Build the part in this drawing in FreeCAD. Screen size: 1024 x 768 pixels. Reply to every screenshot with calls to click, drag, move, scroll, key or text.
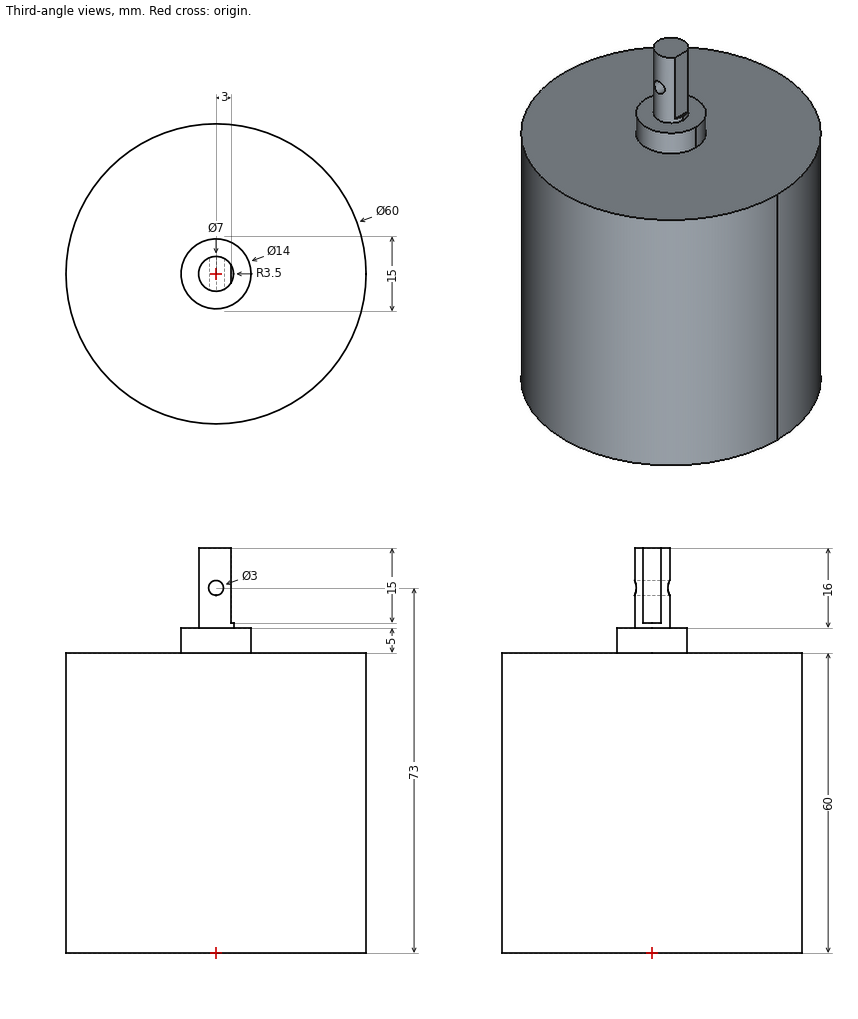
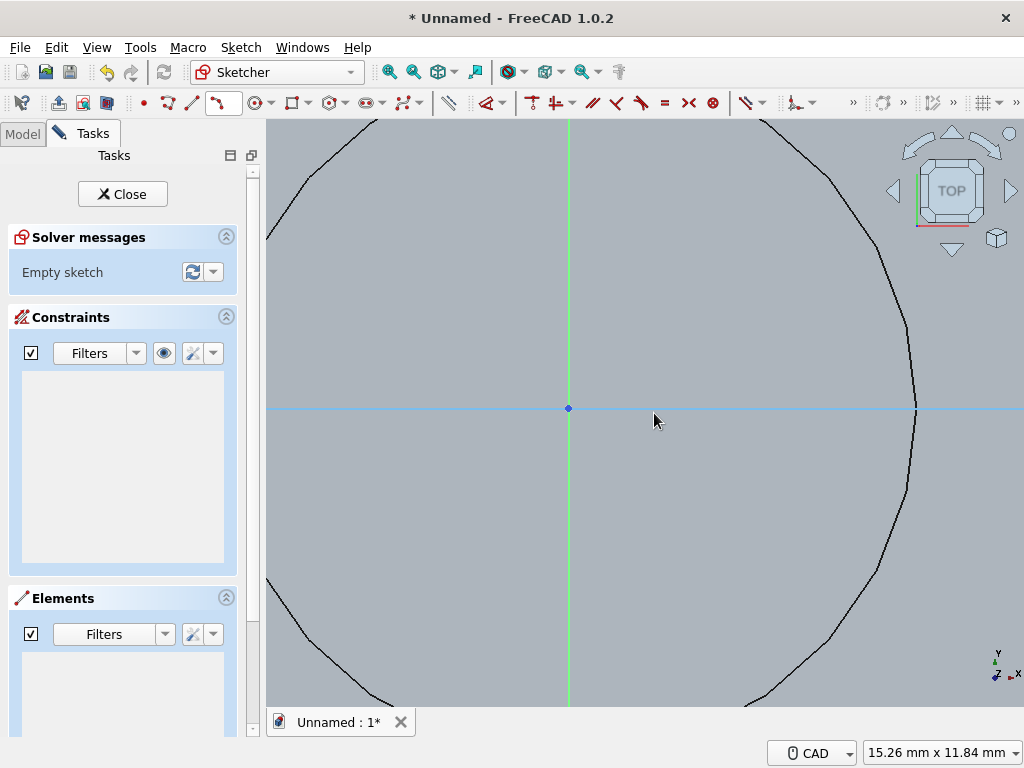
click(256, 104)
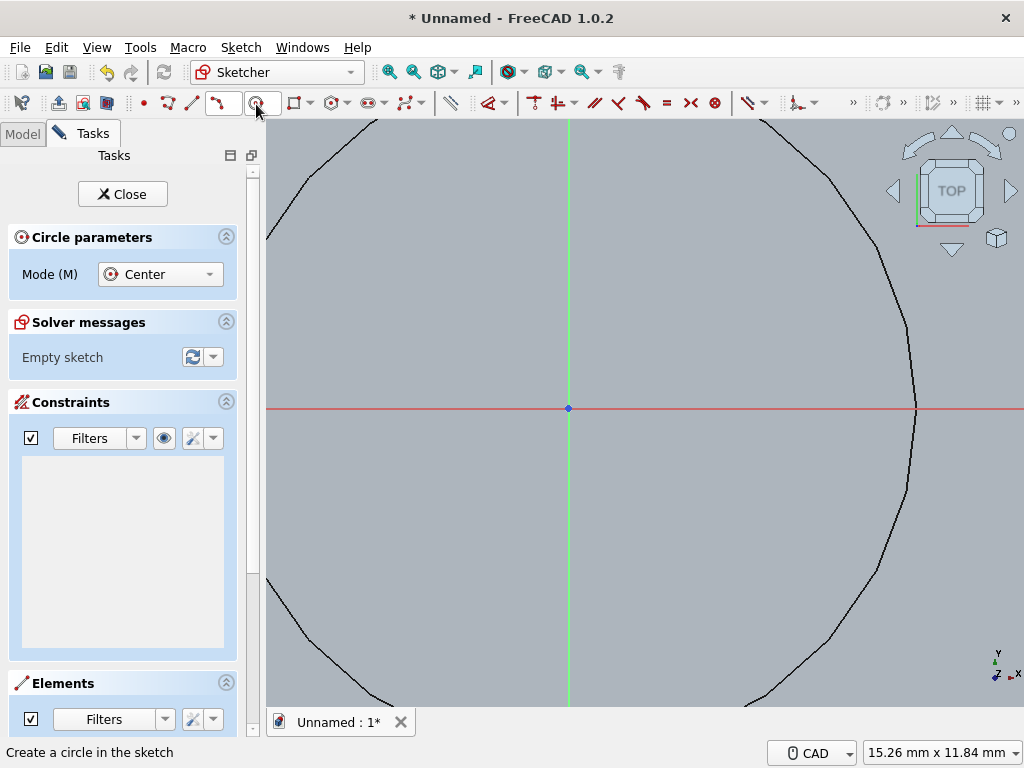
click(569, 409)
move(692, 286)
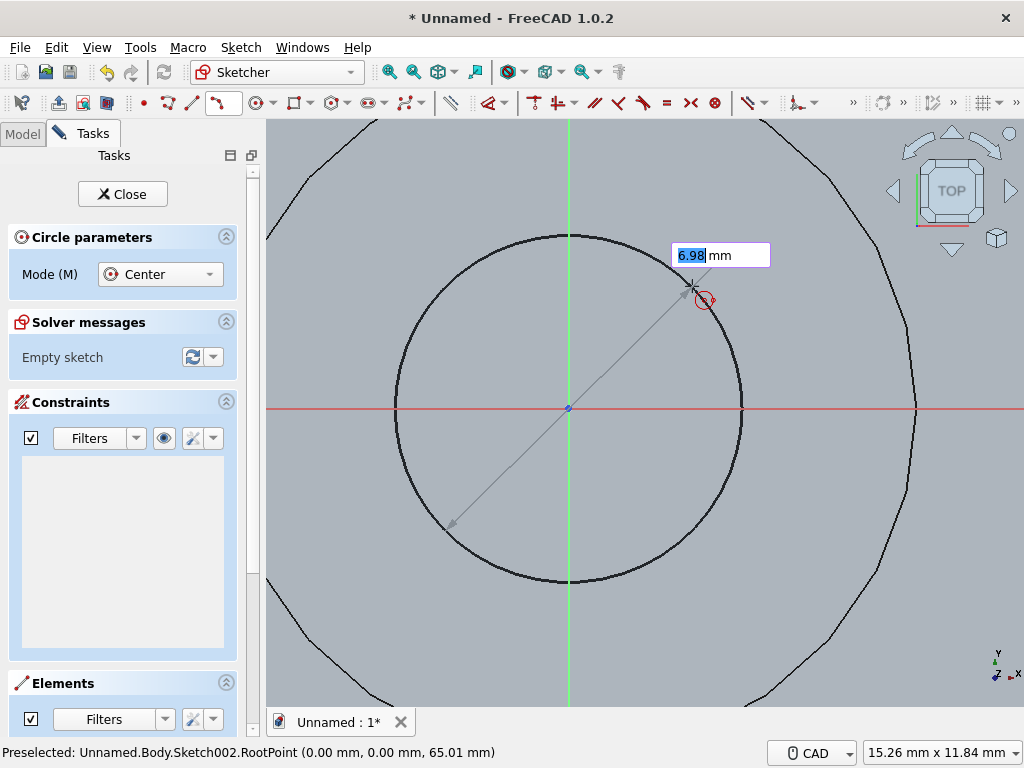
text(7)
key(Return)
key(Escape)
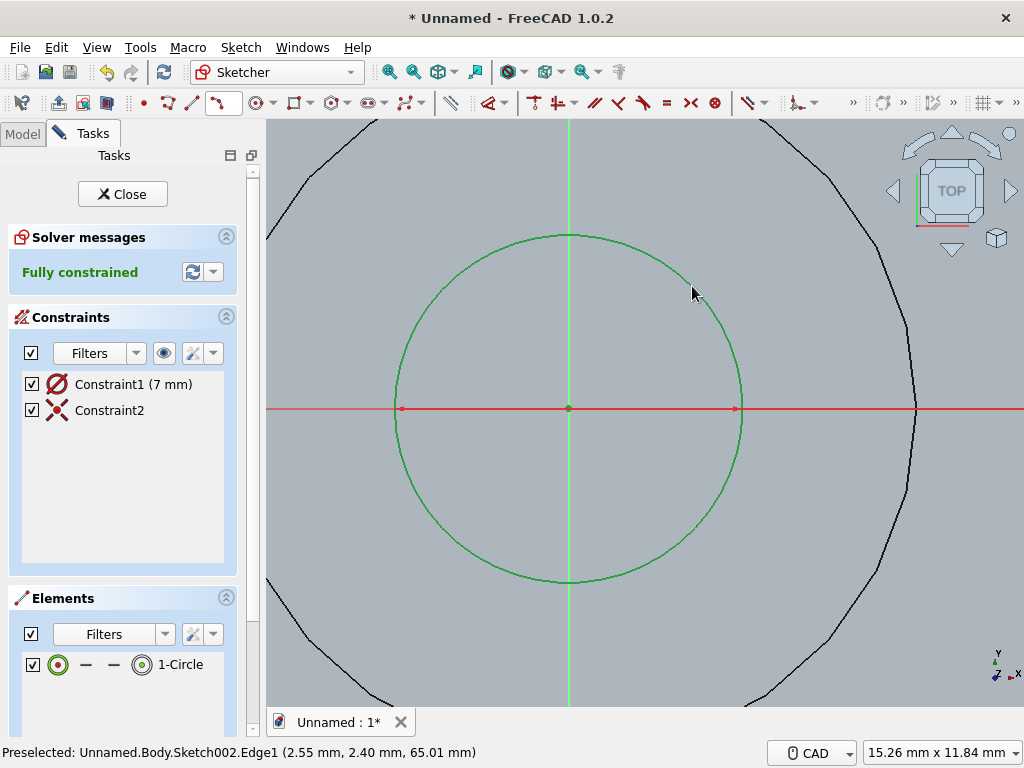
click(123, 194)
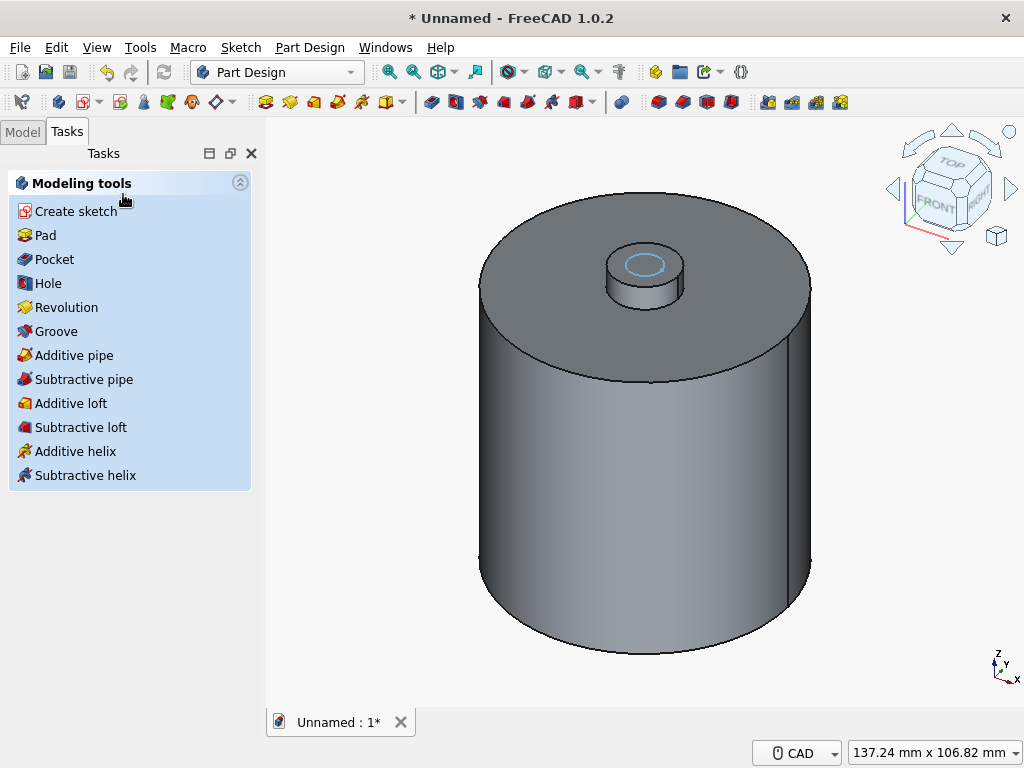
click(266, 102)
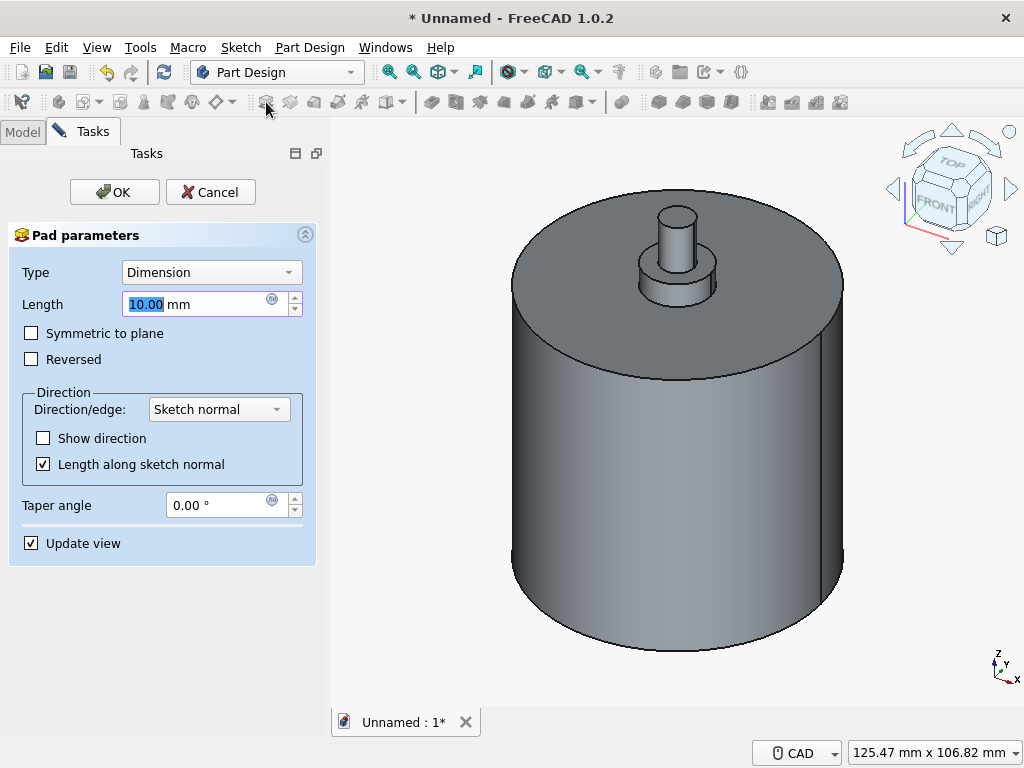
text(16)
key(Tab)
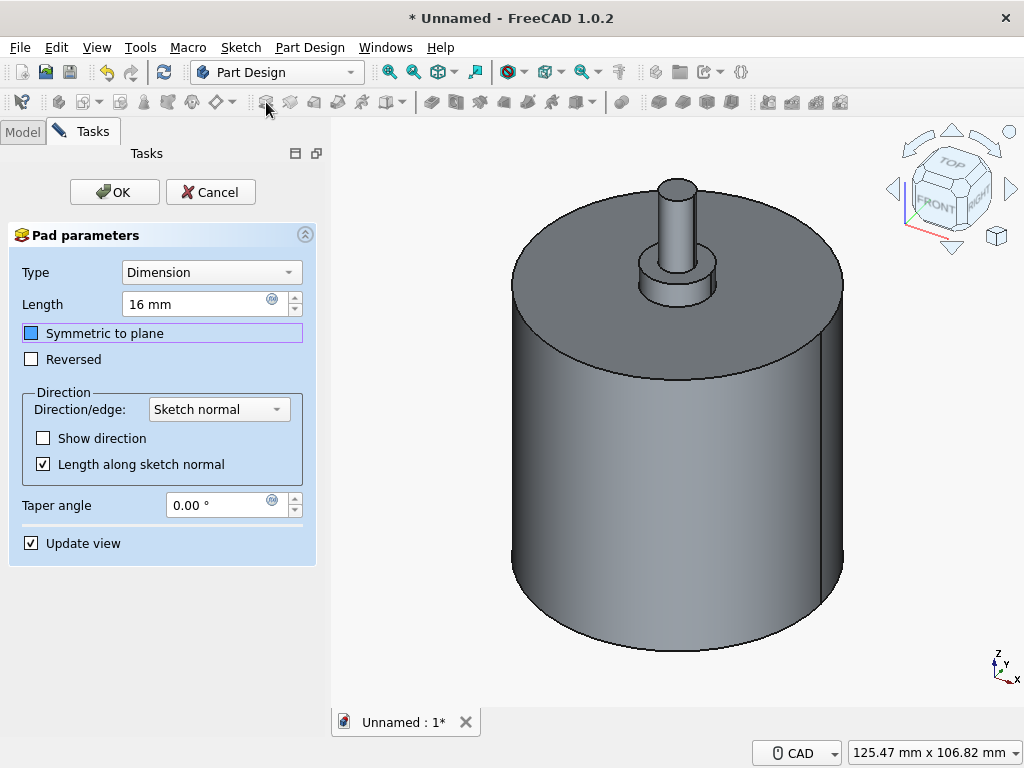
click(115, 192)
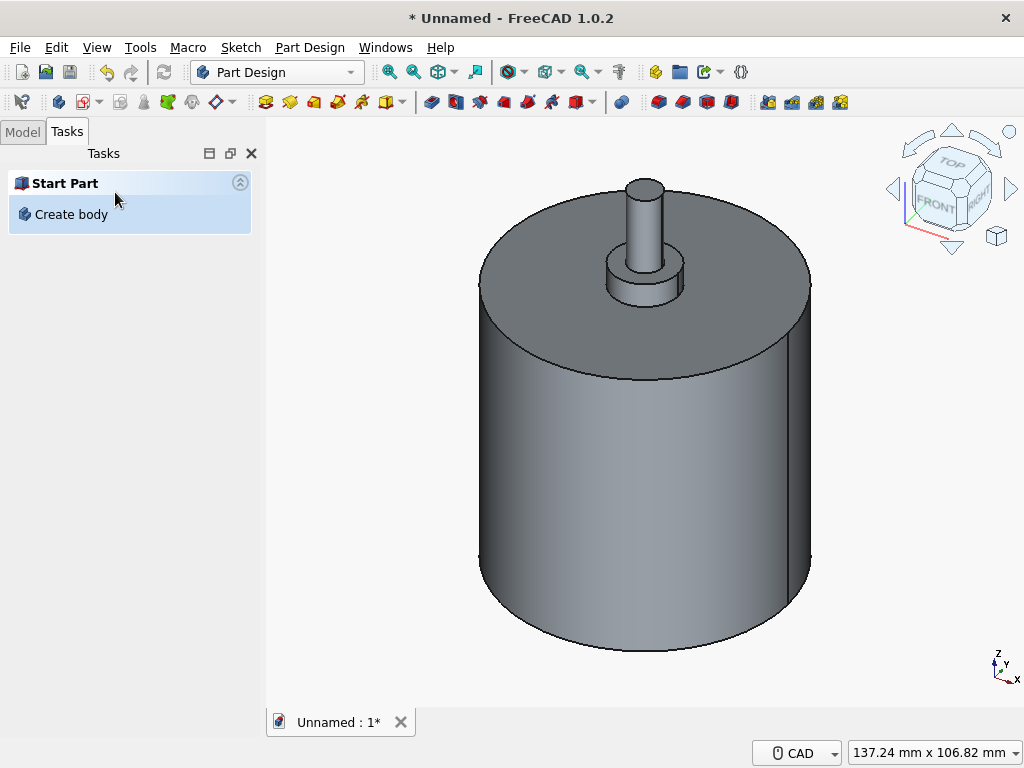
click(390, 72)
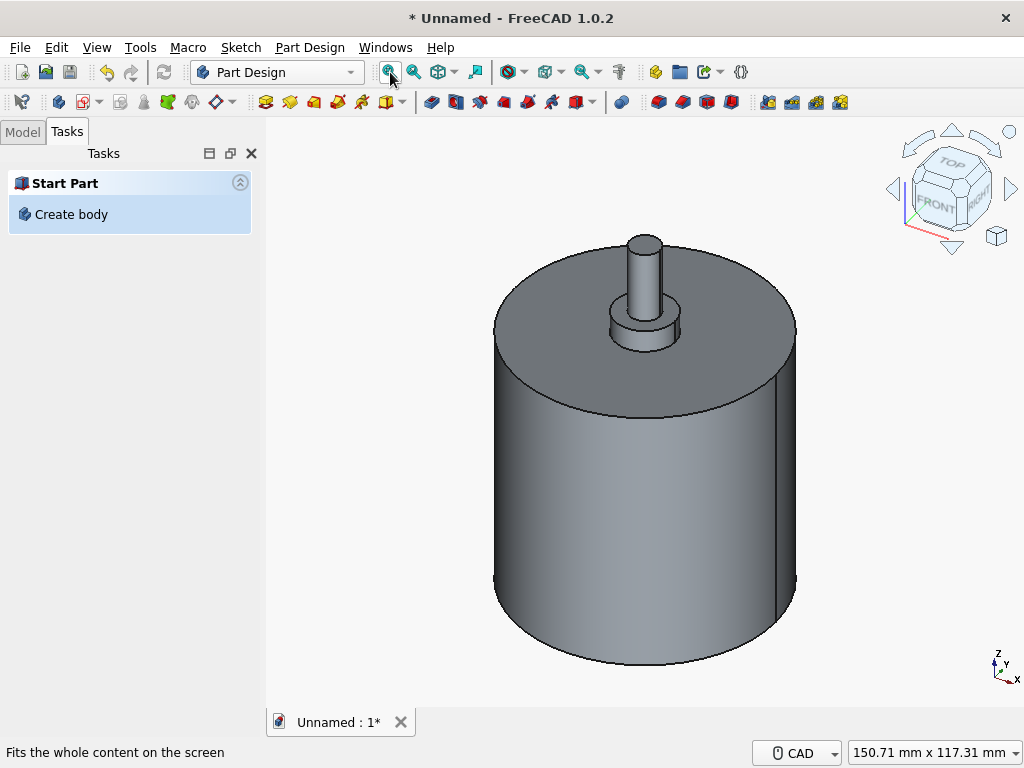
click(23, 131)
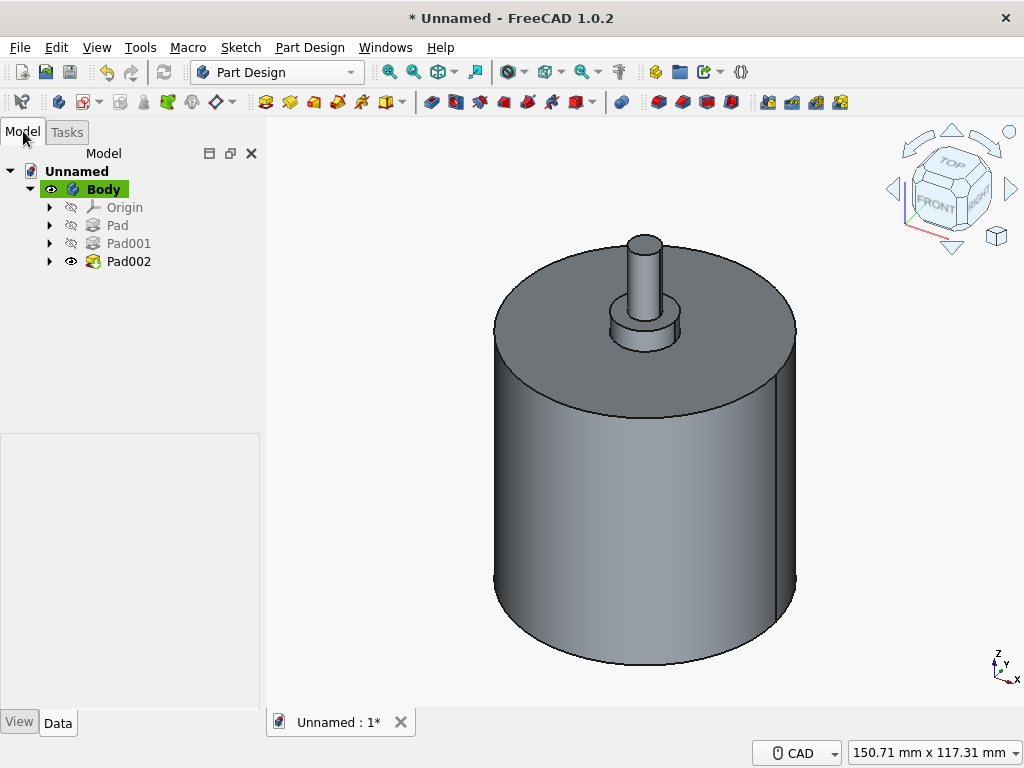
click(50, 207)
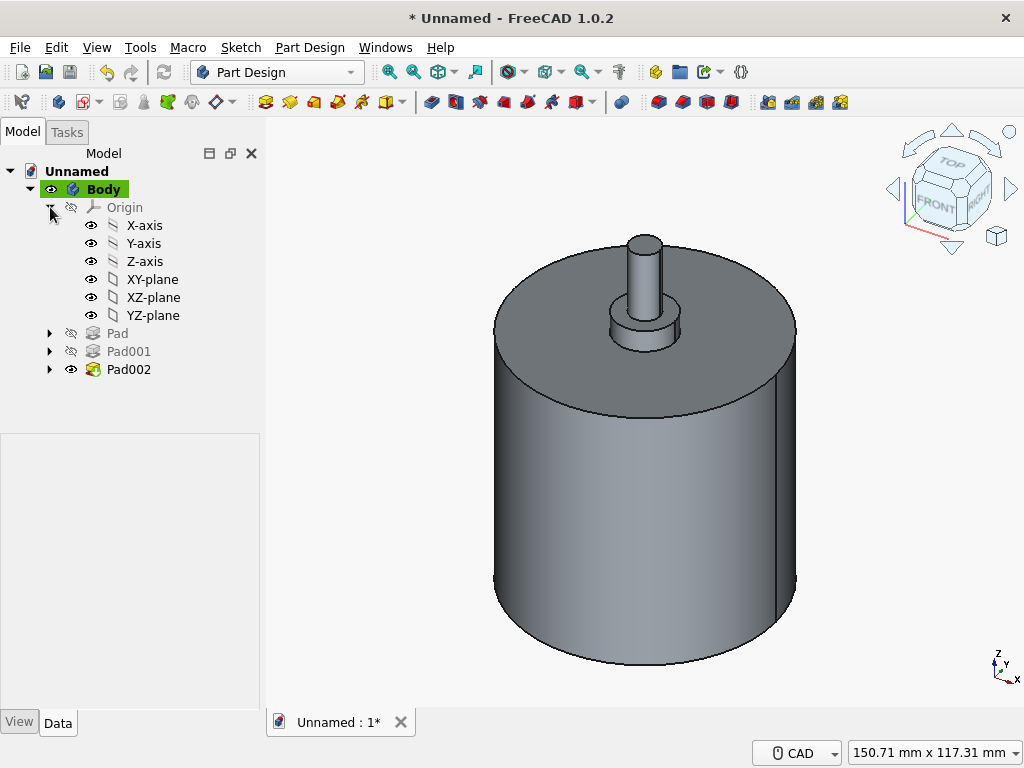
click(136, 279)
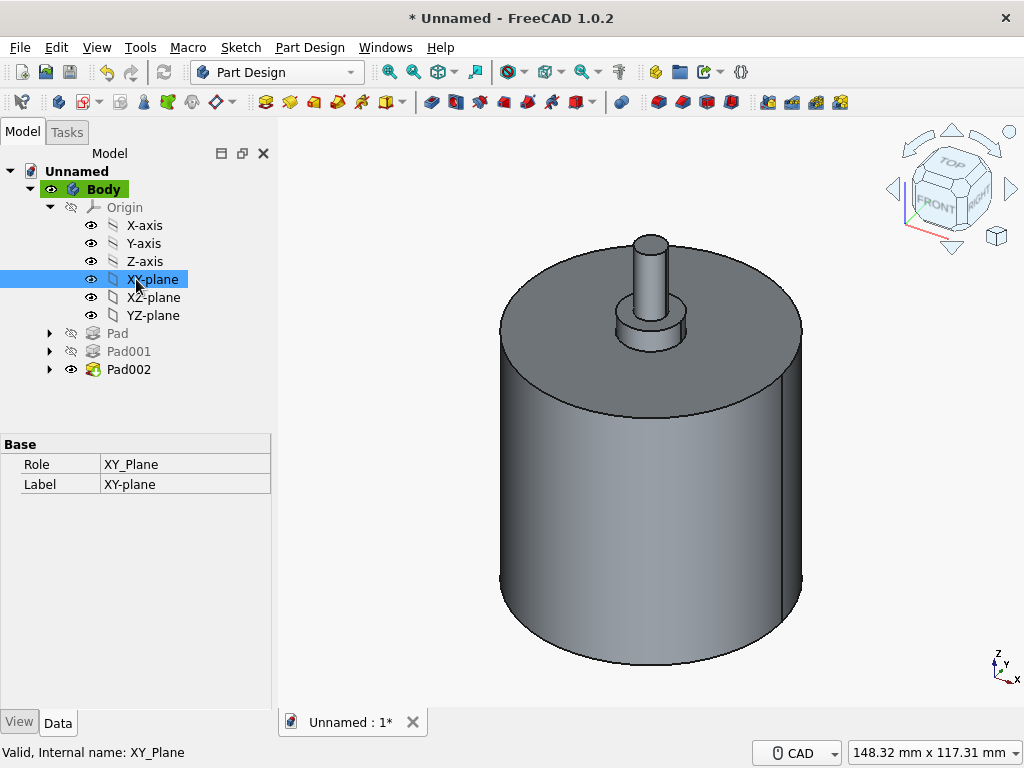
click(216, 102)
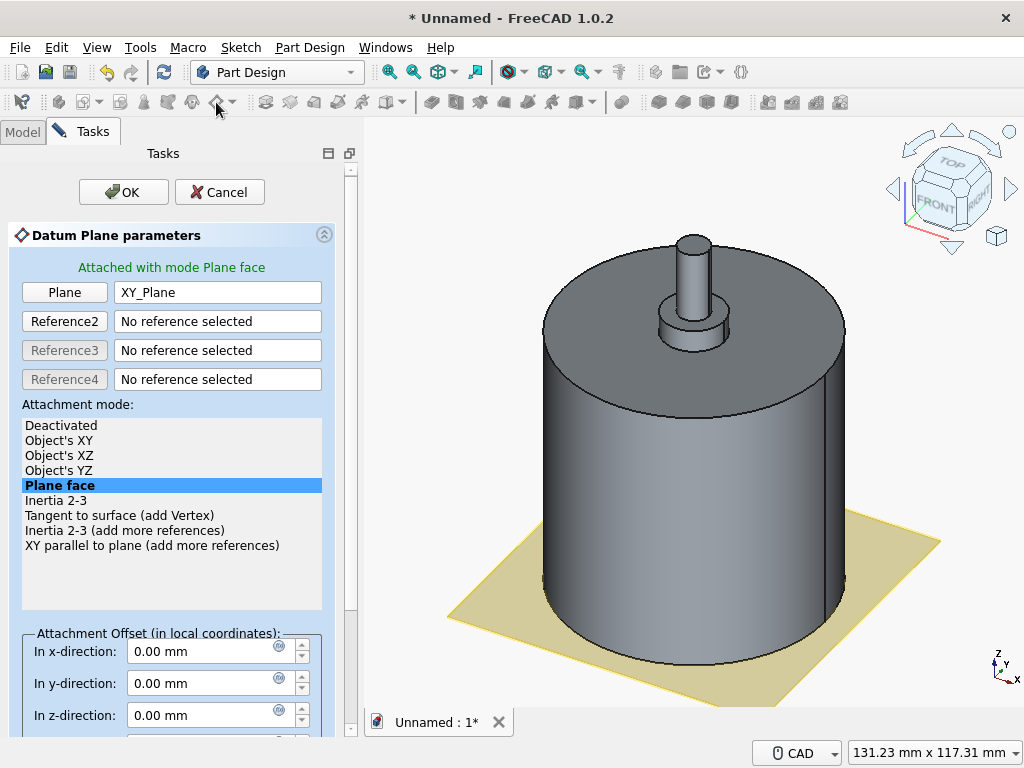
triple_click(210, 715)